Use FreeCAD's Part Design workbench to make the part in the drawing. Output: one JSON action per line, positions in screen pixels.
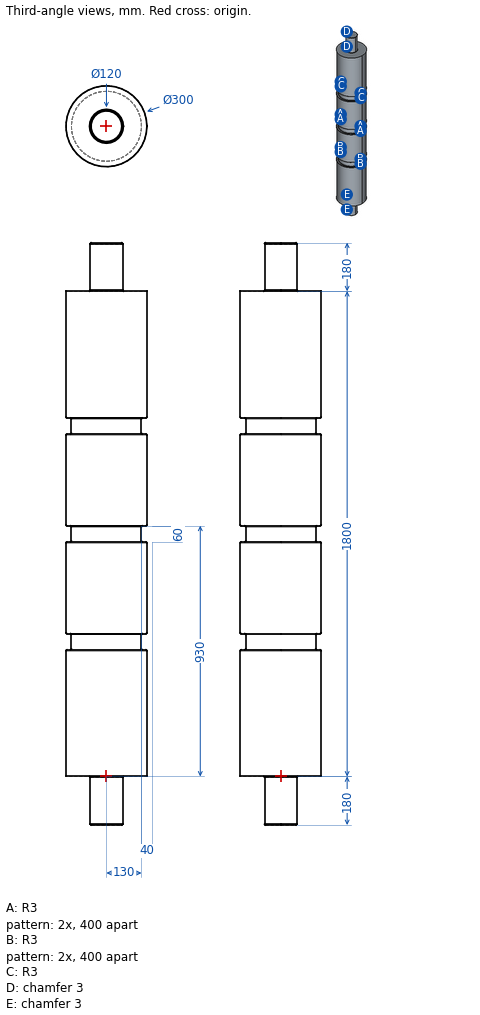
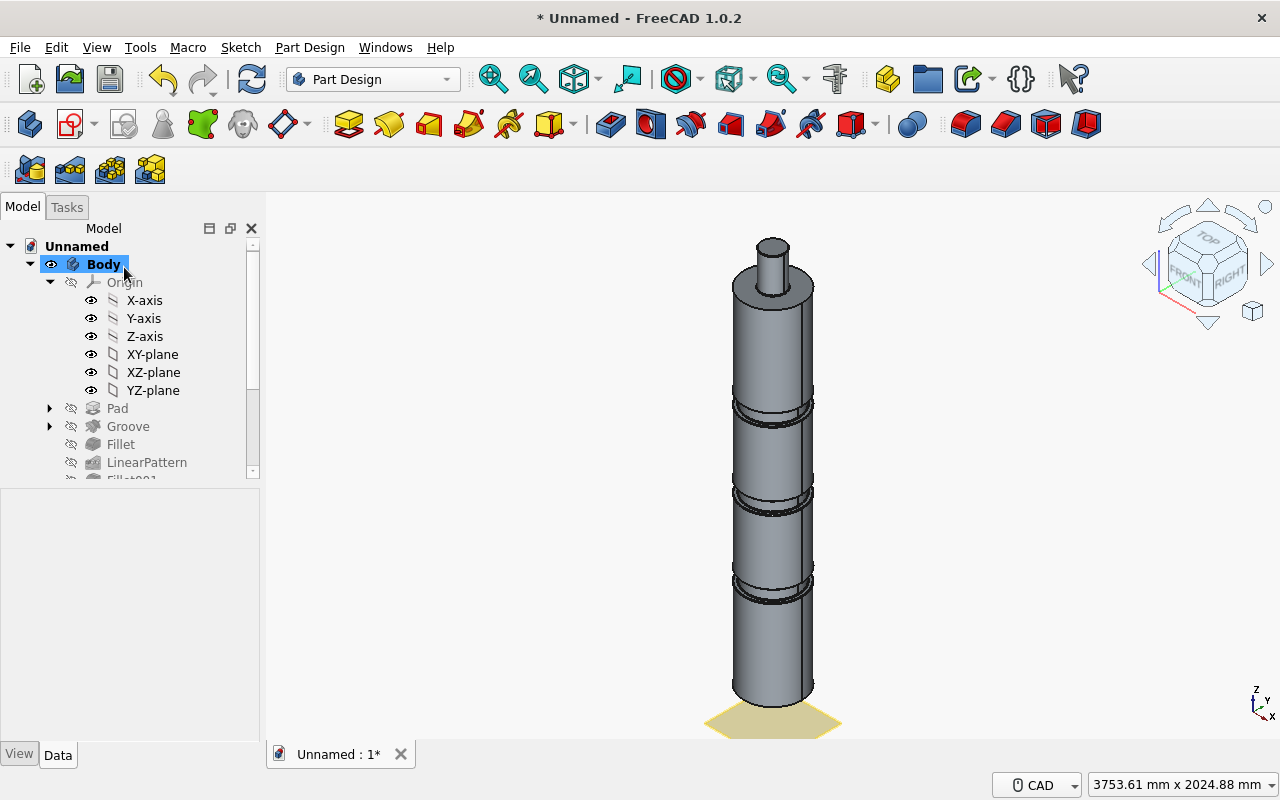
{"action": "scroll", "coordinate": [100, 350], "scroll_direction": "down", "scroll_amount": 3}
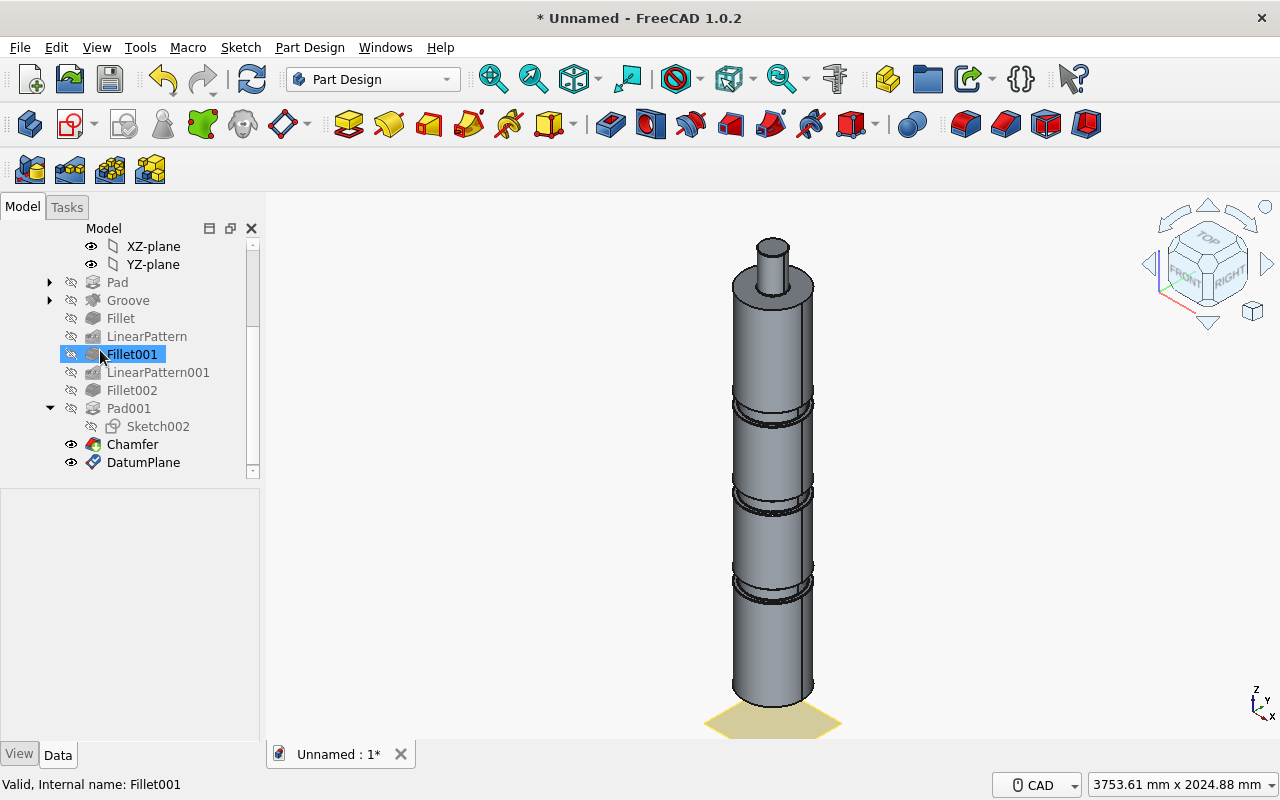
{"action": "left_click", "coordinate": [116, 462]}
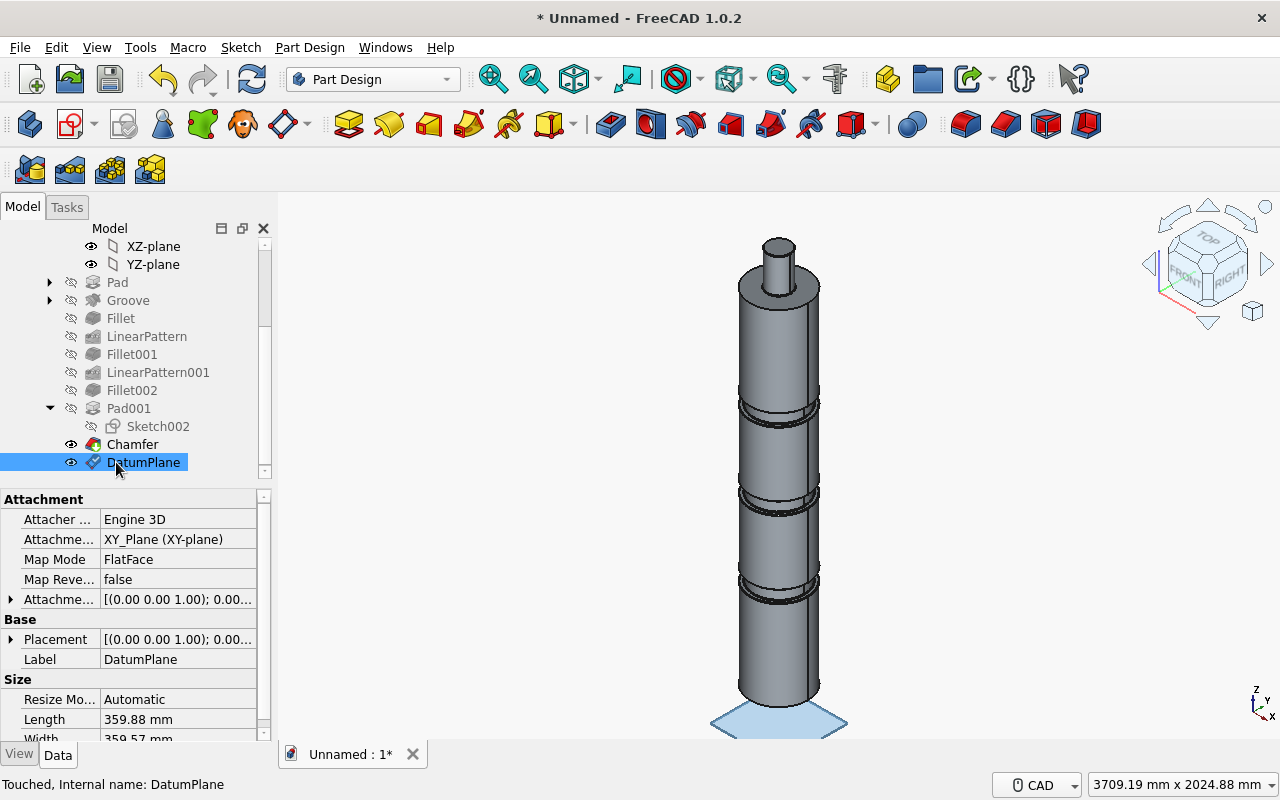
{"action": "left_click", "coordinate": [70, 124]}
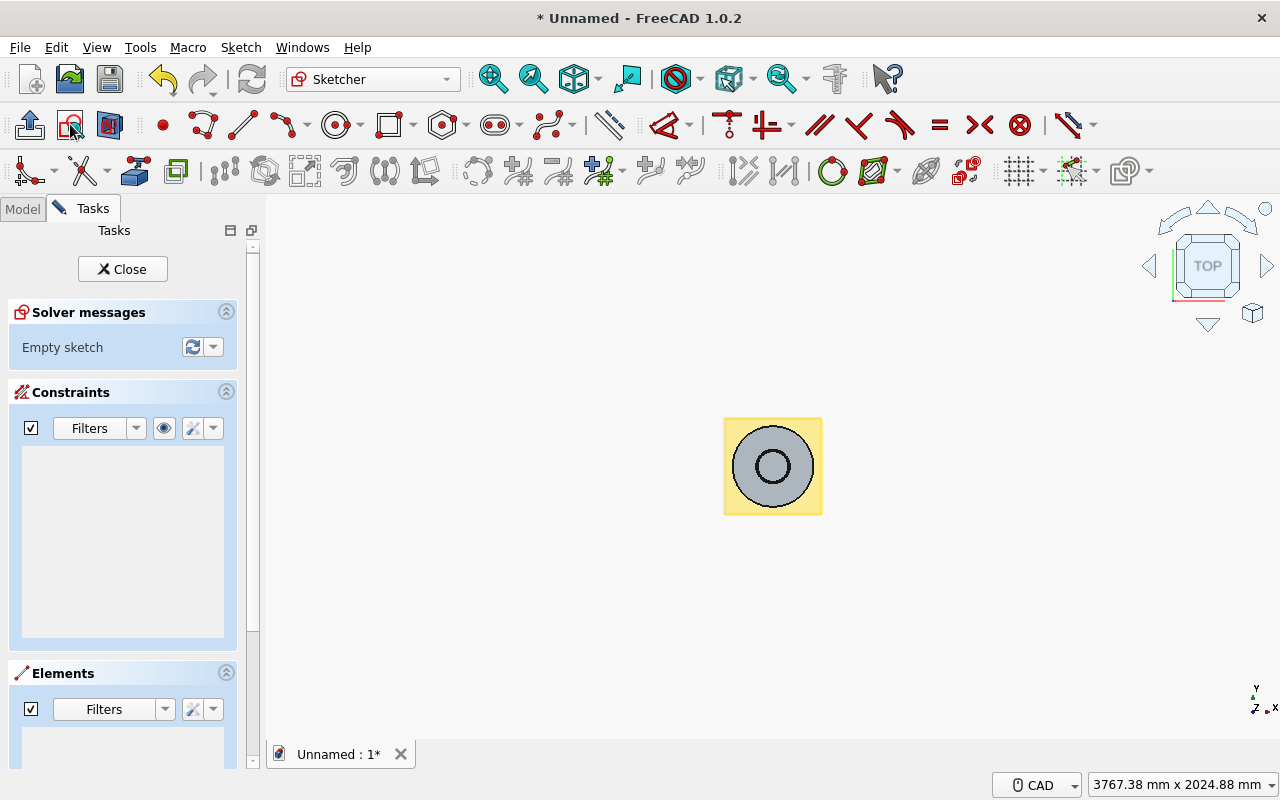
{"action": "left_click", "coordinate": [110, 126]}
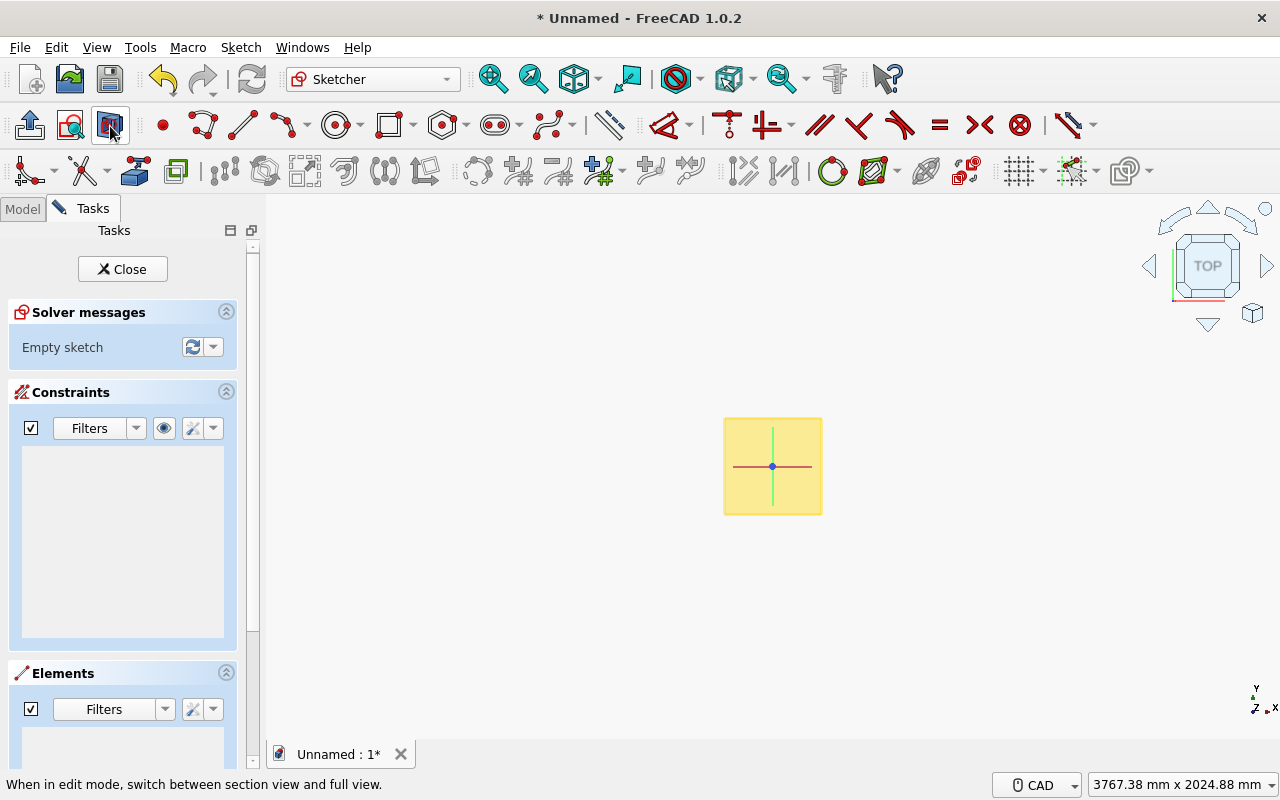
{"action": "scroll", "coordinate": [780, 467], "scroll_direction": "up", "scroll_amount": 12}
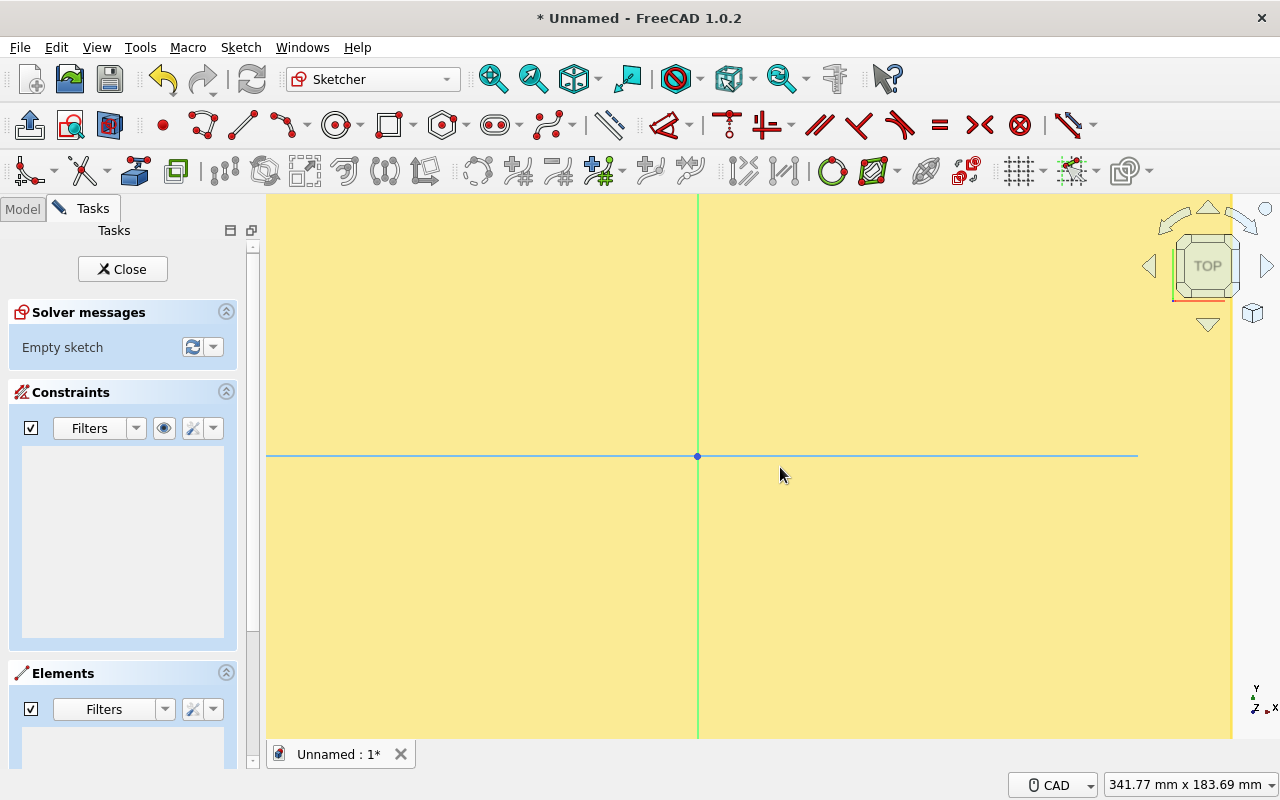
{"action": "key", "text": "g c"}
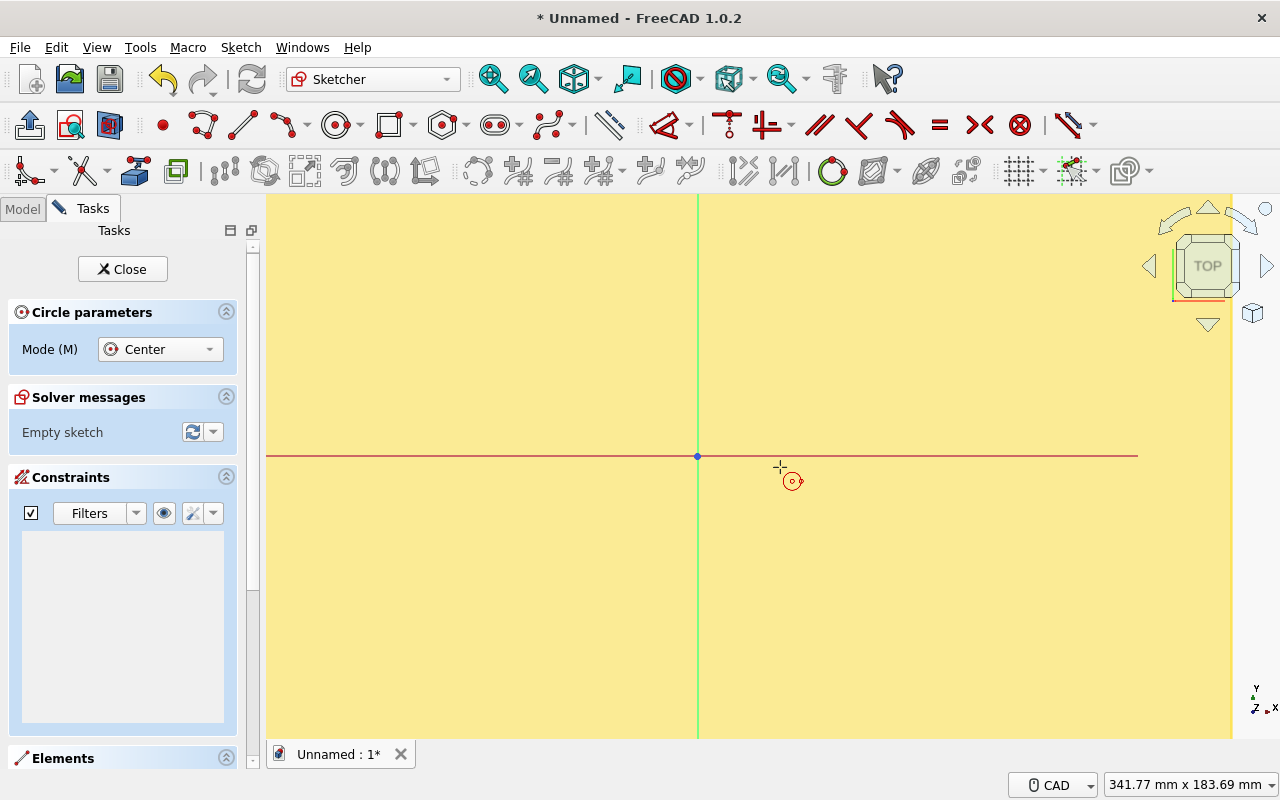
{"action": "left_click", "coordinate": [698, 456]}
{"action": "mouse_move", "coordinate": [824, 331]}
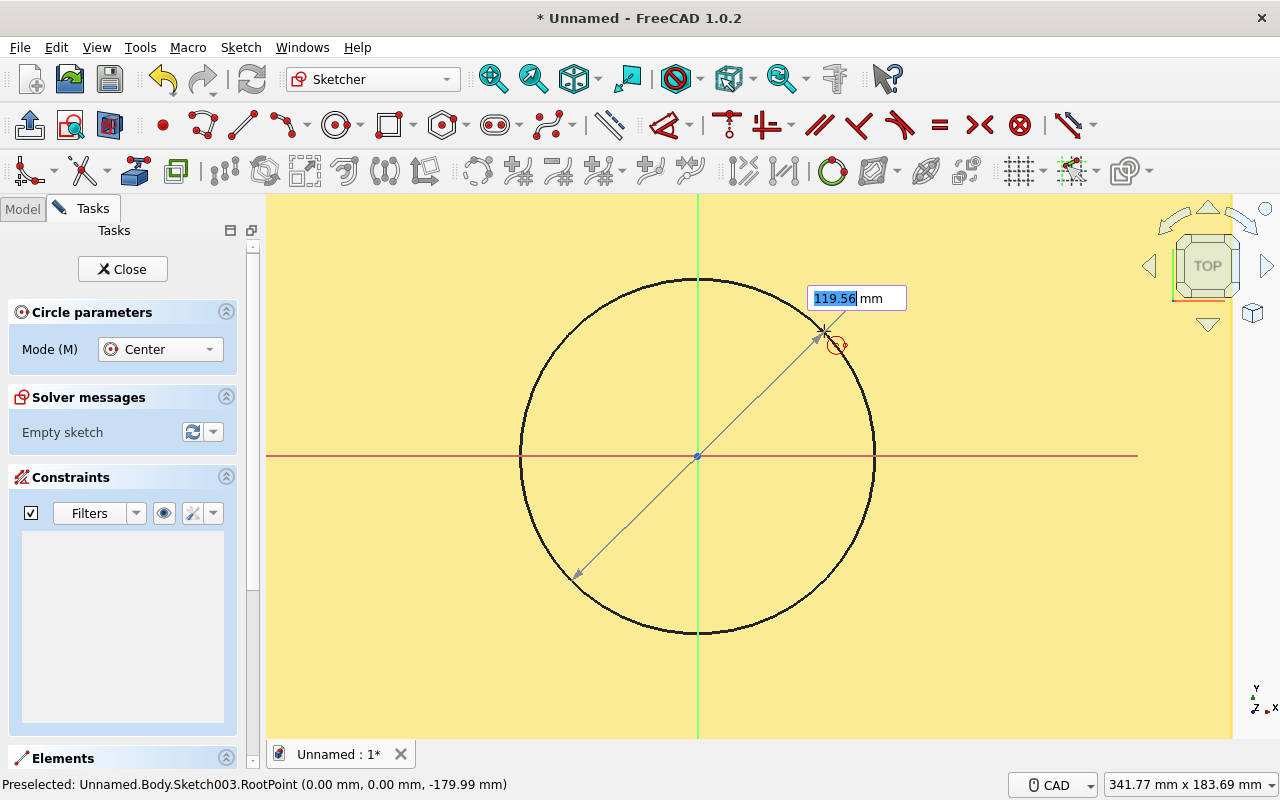
{"action": "type", "text": "120"}
{"action": "key", "text": "Return"}
{"action": "key", "text": "Escape"}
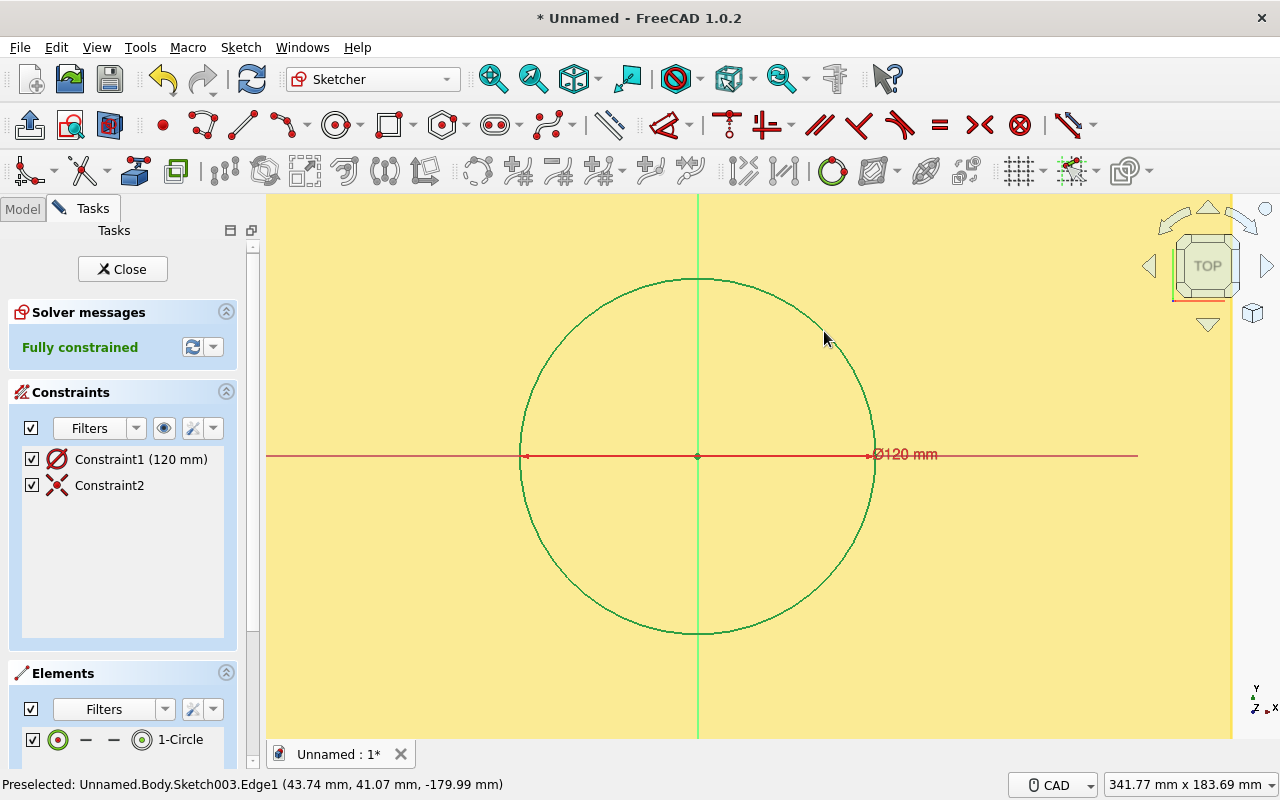
{"action": "left_click", "coordinate": [123, 269]}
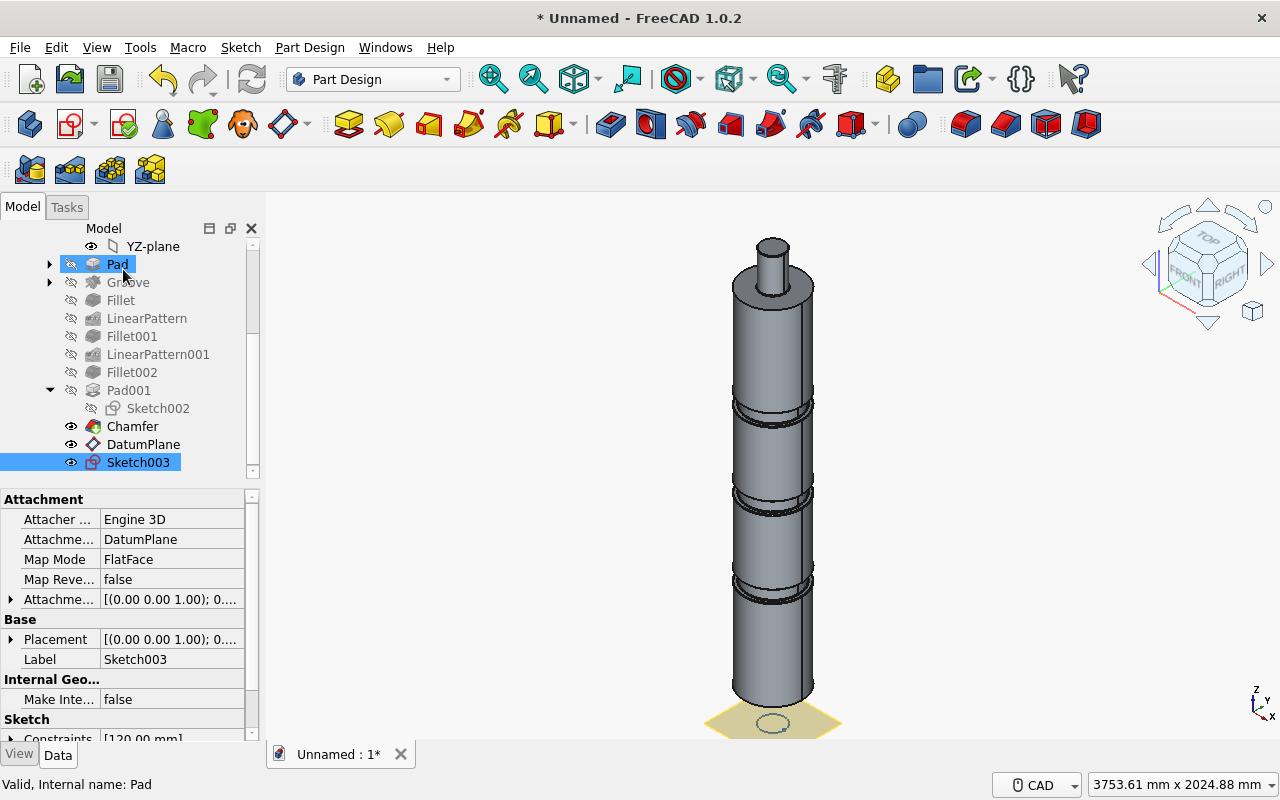
{"action": "left_click", "coordinate": [350, 124]}